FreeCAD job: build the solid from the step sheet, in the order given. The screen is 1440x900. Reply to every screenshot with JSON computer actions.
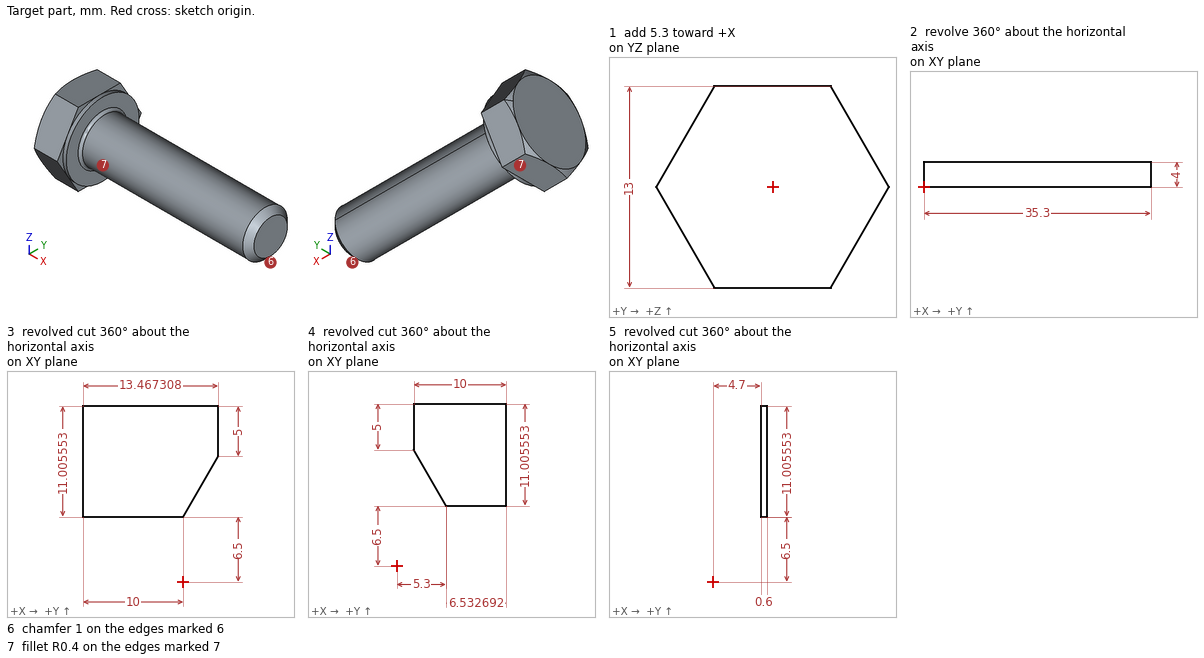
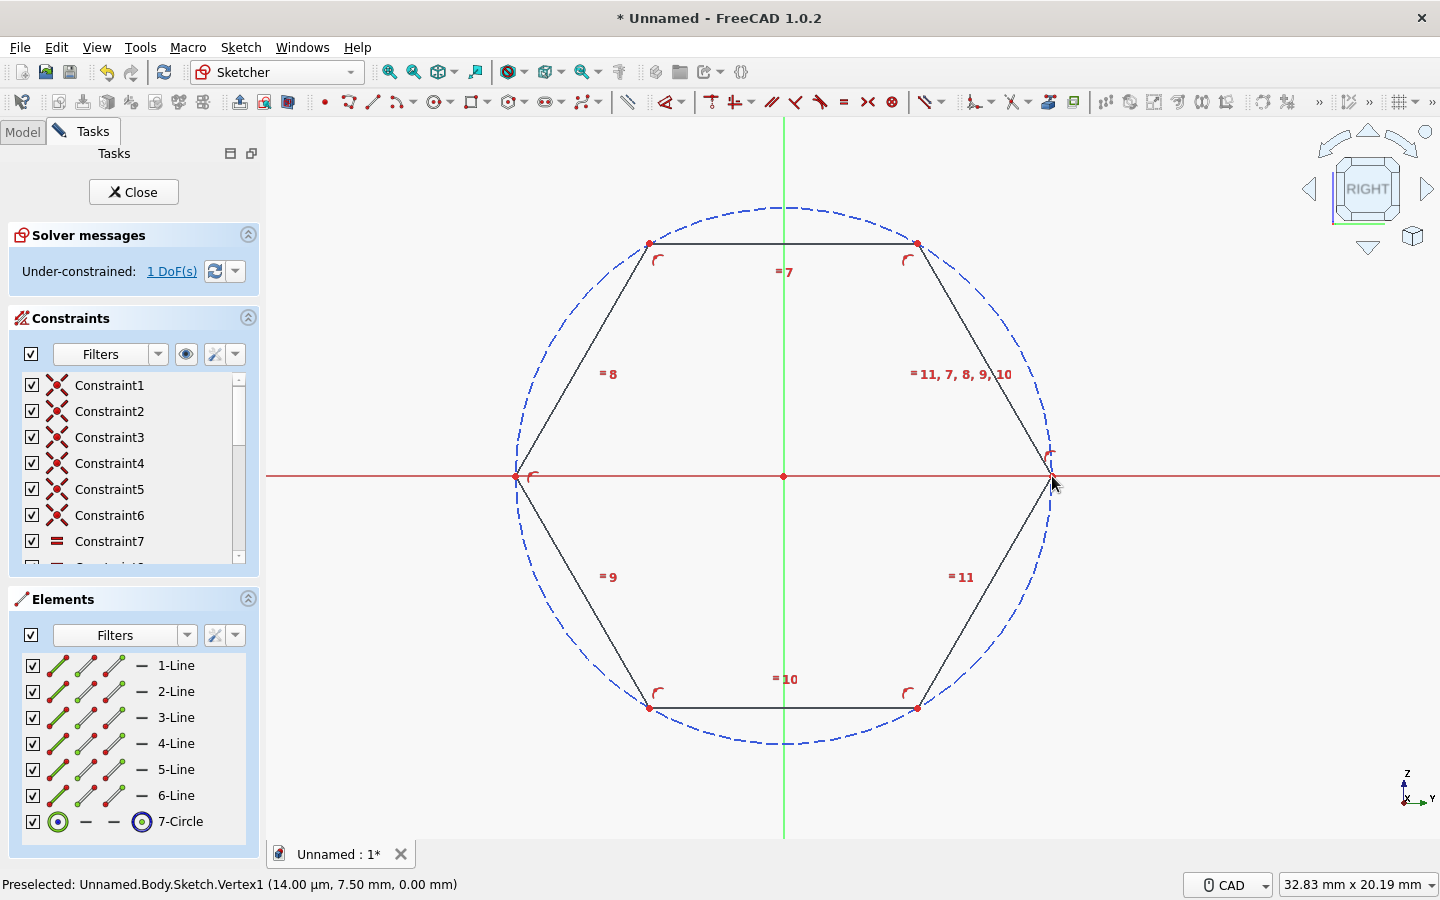
{"action": "key", "text": "d"}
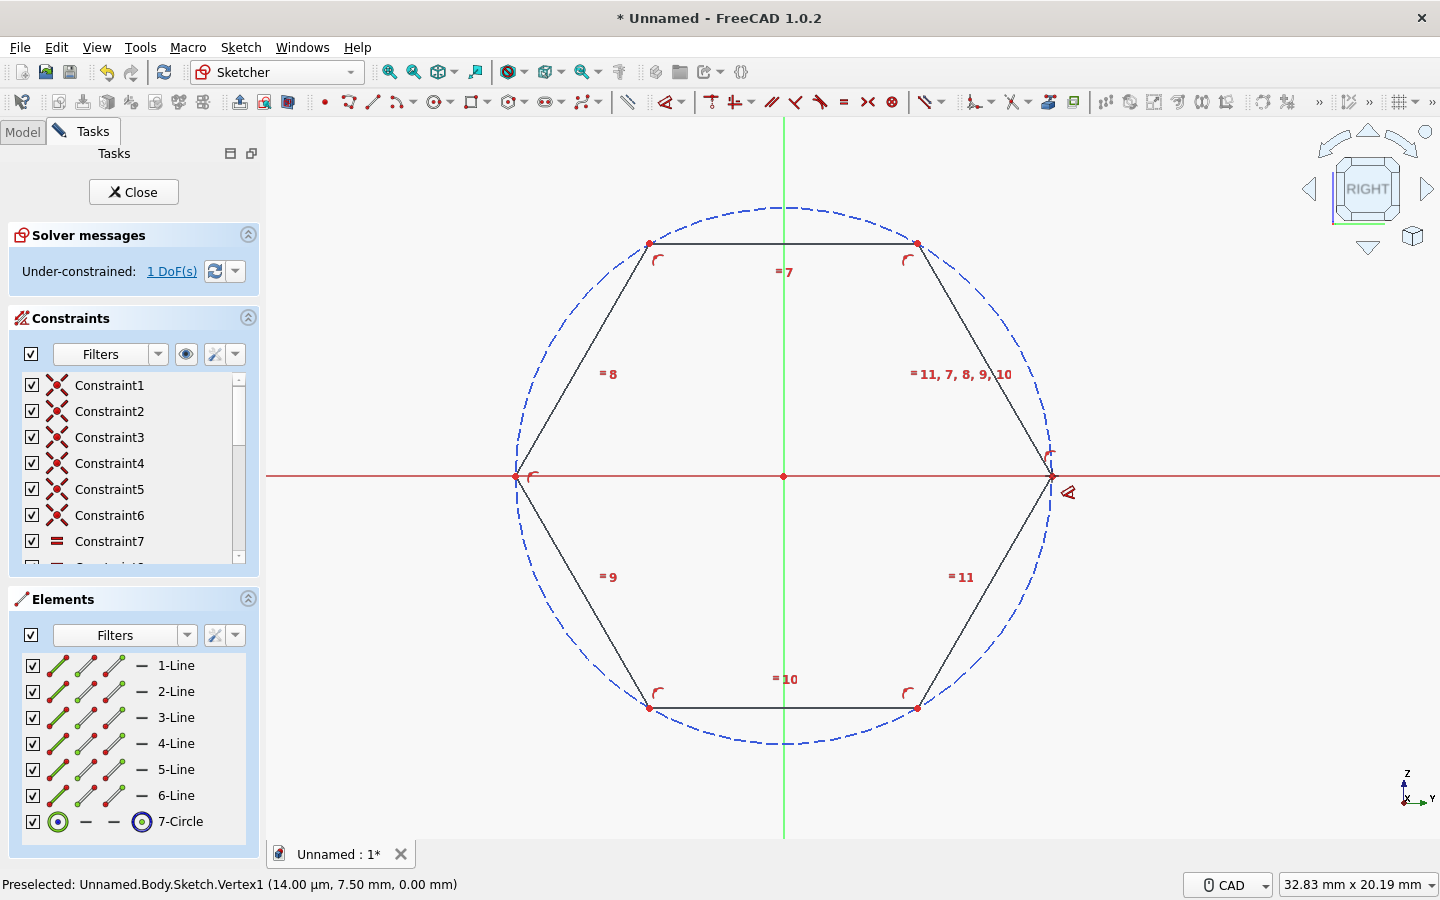
{"action": "left_click", "coordinate": [650, 708]}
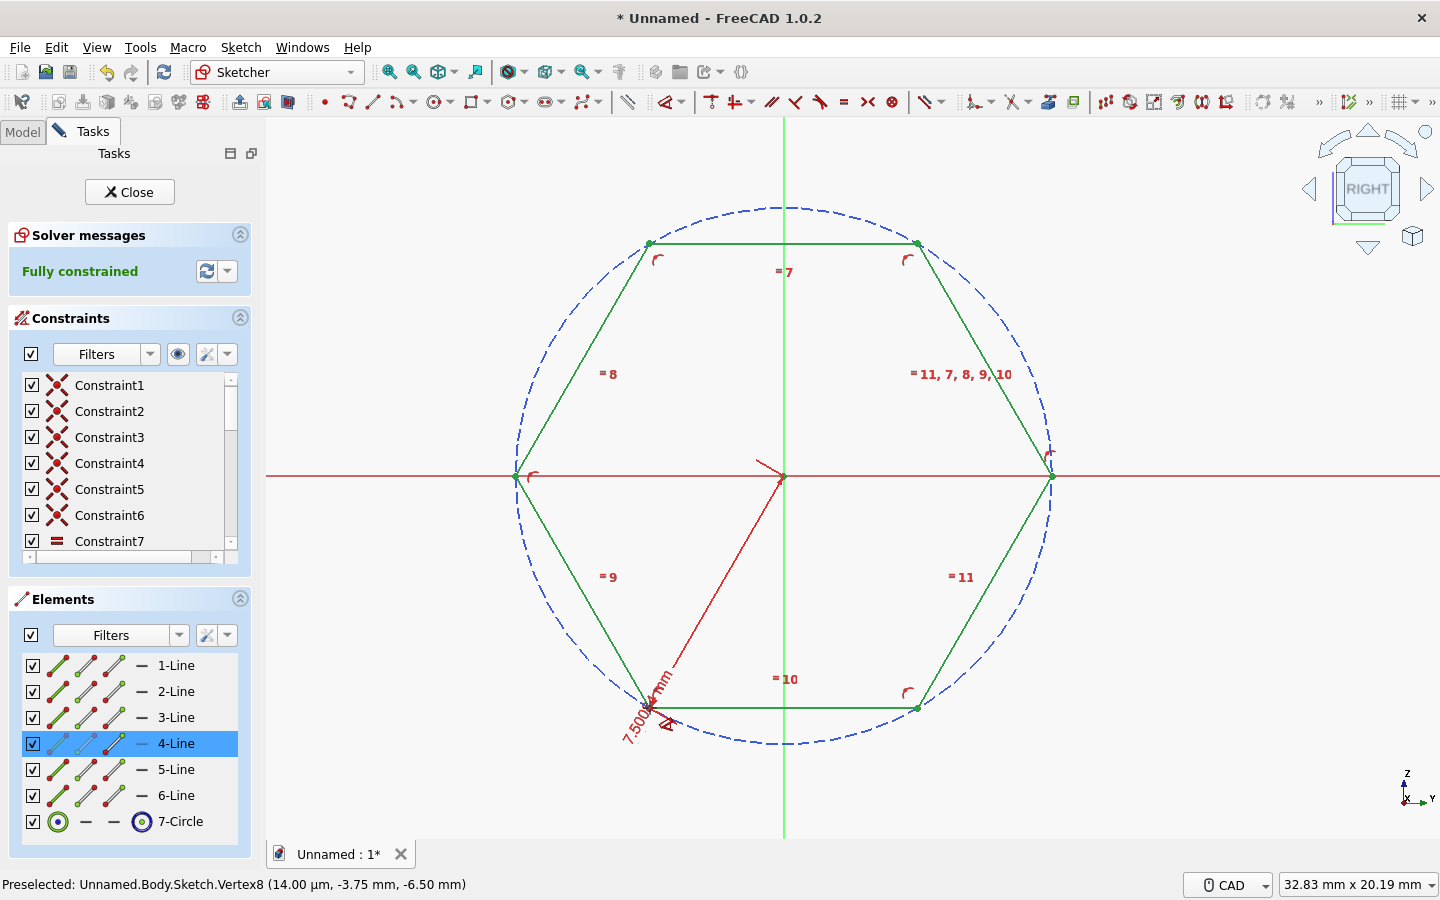
{"action": "left_click", "coordinate": [918, 244]}
{"action": "left_click", "coordinate": [952, 369]}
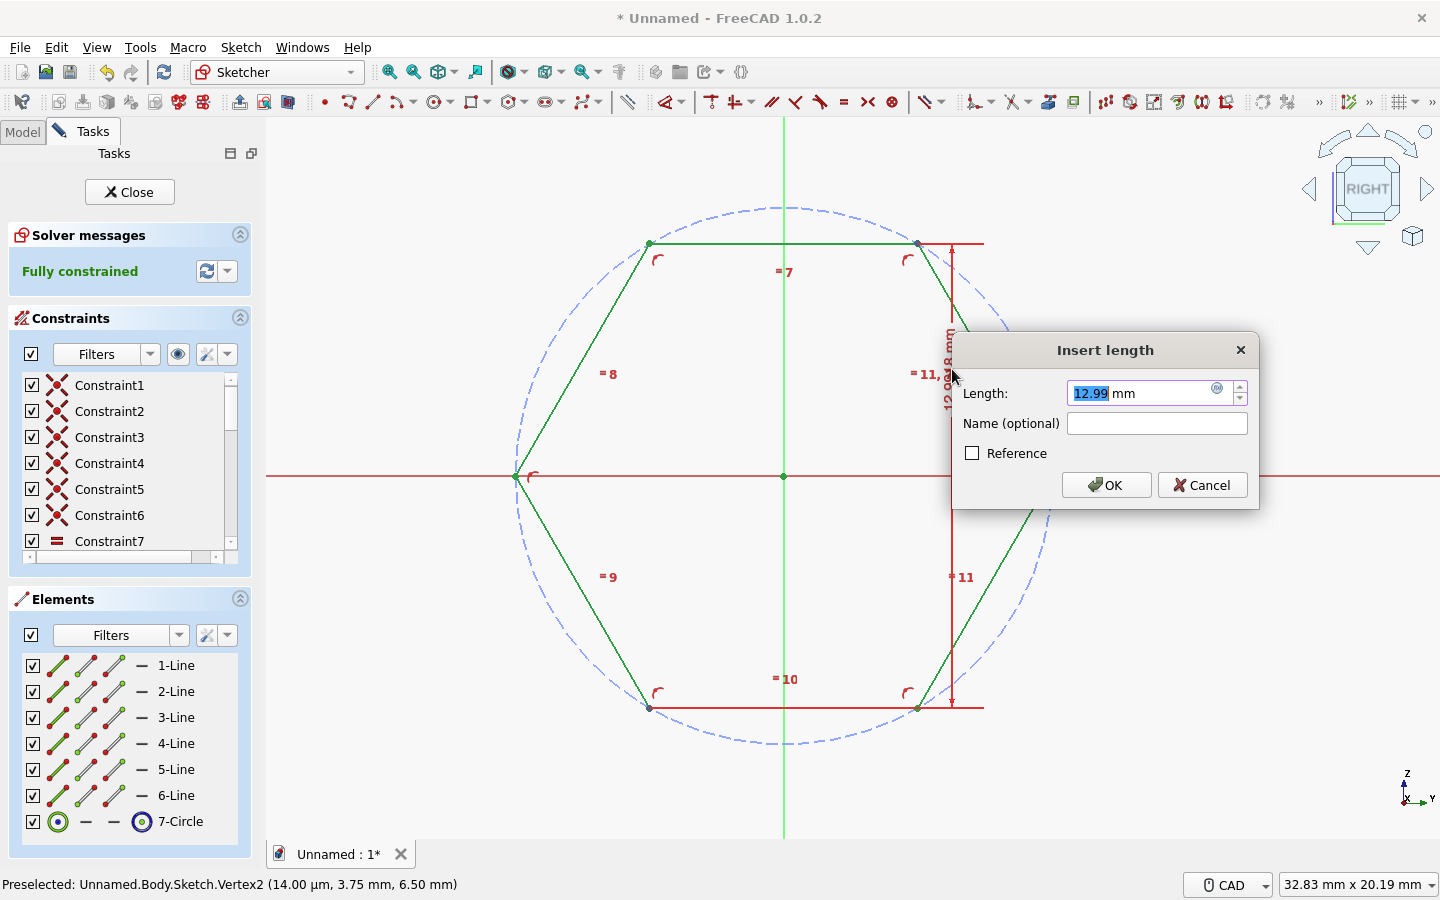
{"action": "type", "text": "13"}
{"action": "key", "text": "Return"}
{"action": "key", "text": "Escape"}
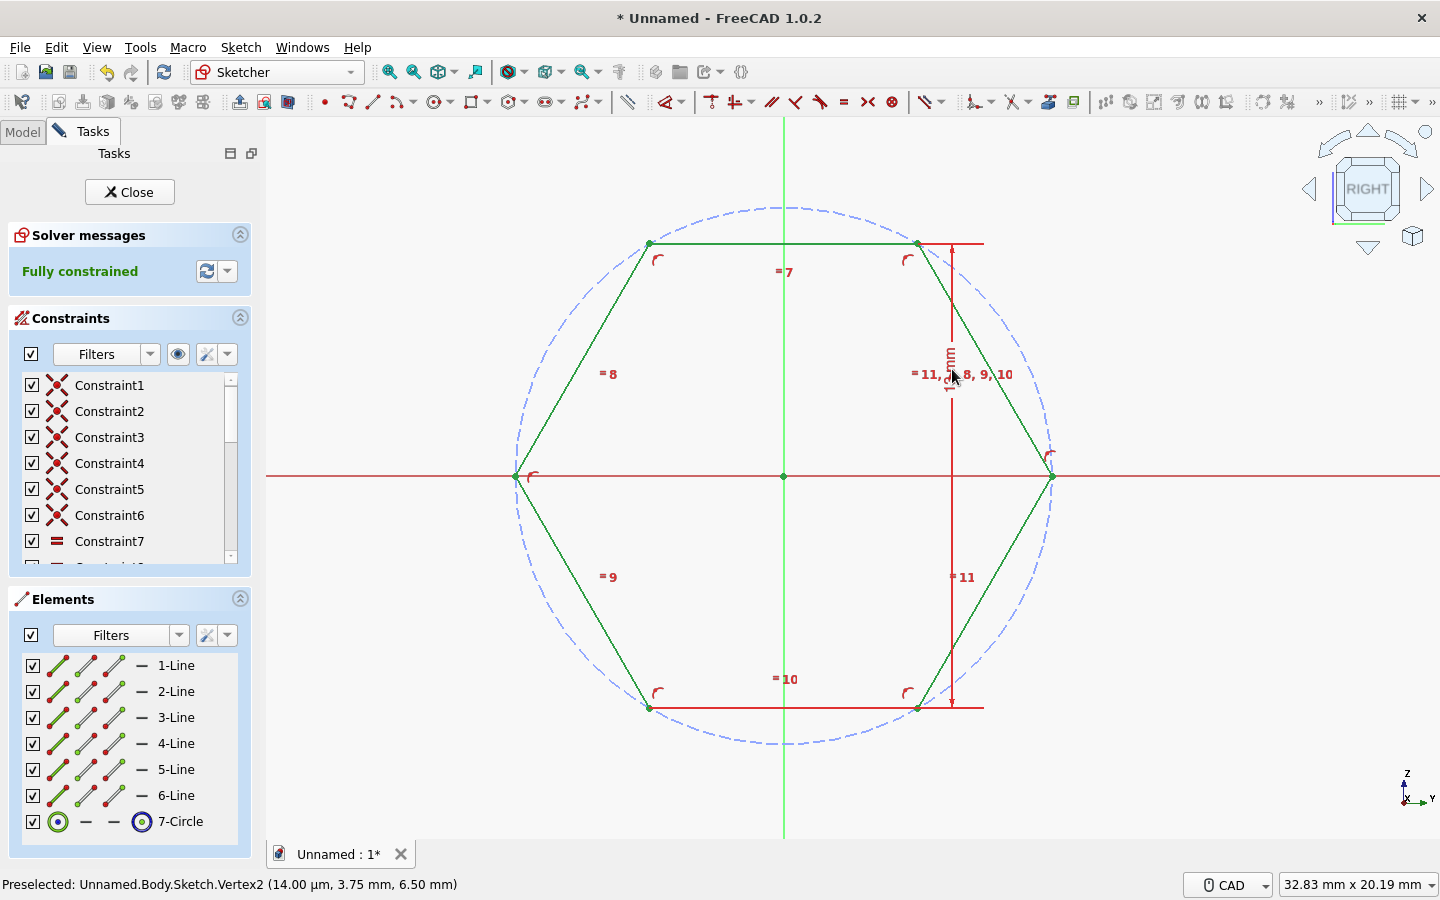
{"action": "left_click", "coordinate": [130, 192]}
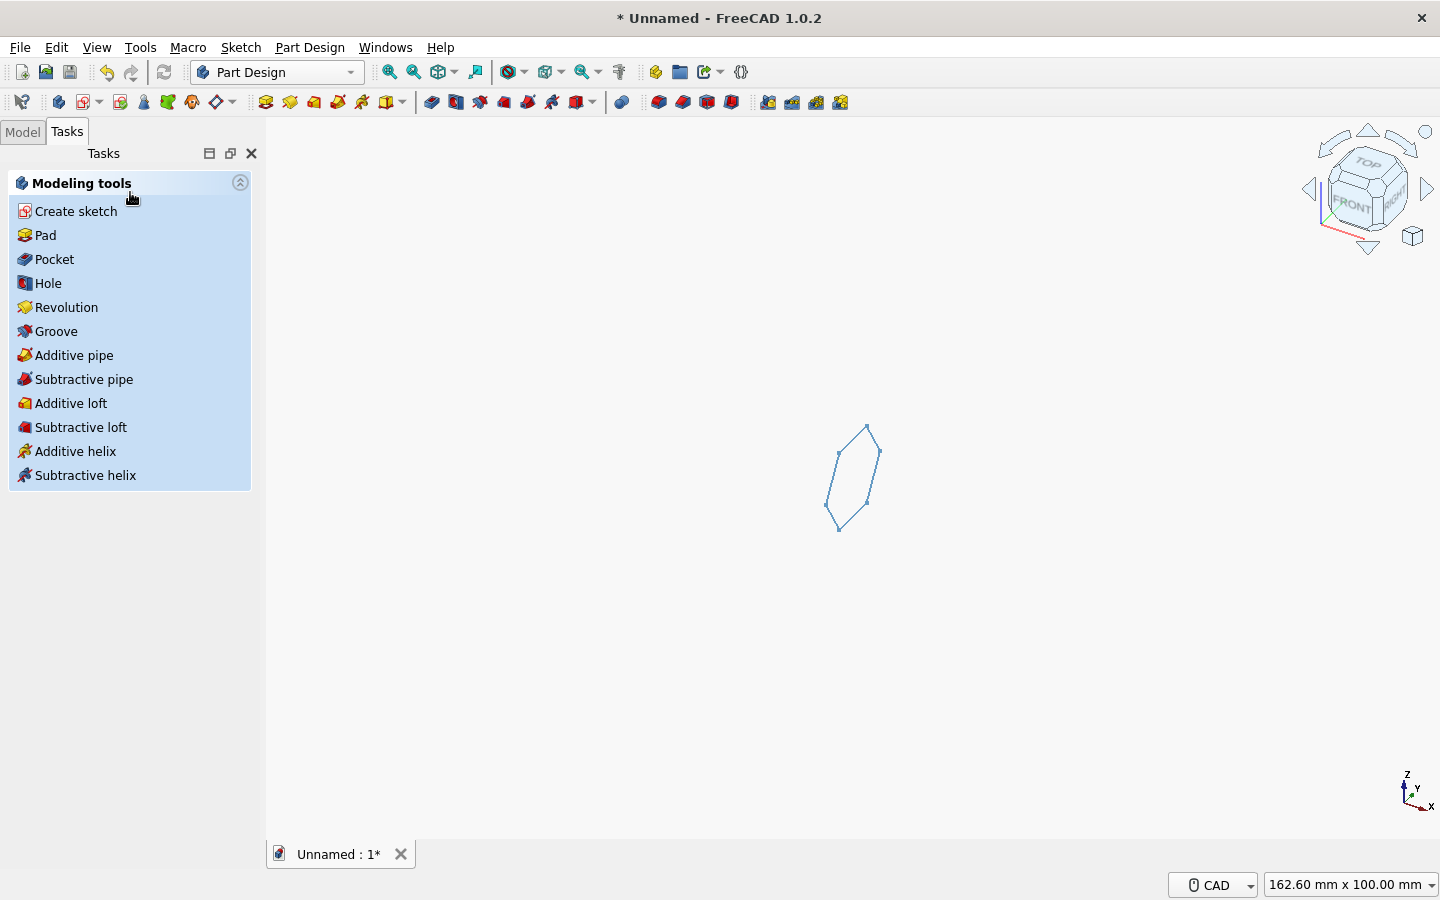
{"action": "left_click", "coordinate": [266, 102]}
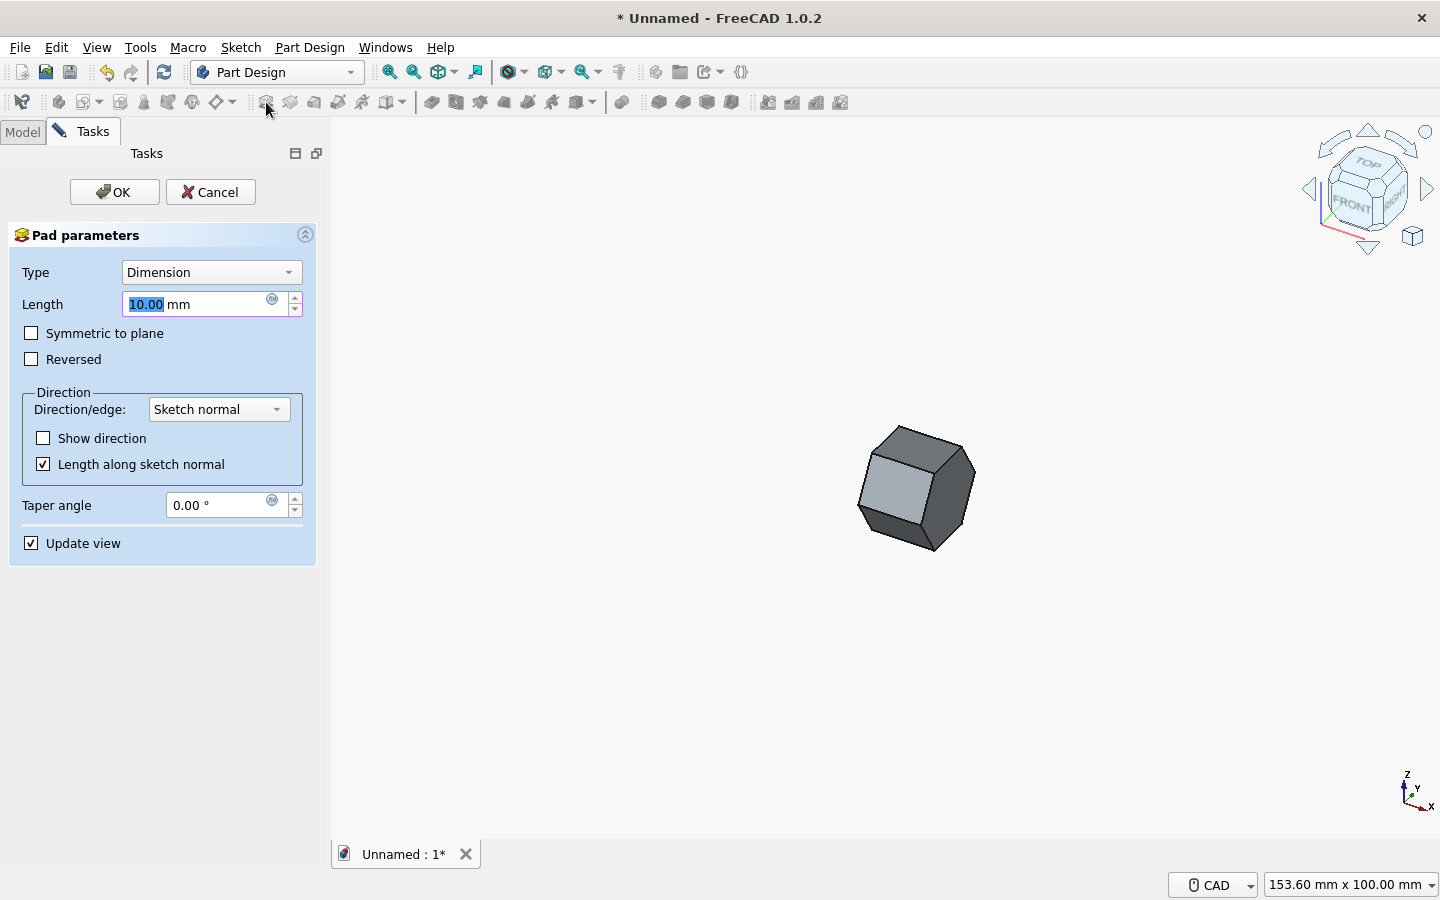
{"action": "type", "text": "5.3"}
{"action": "key", "text": "Tab"}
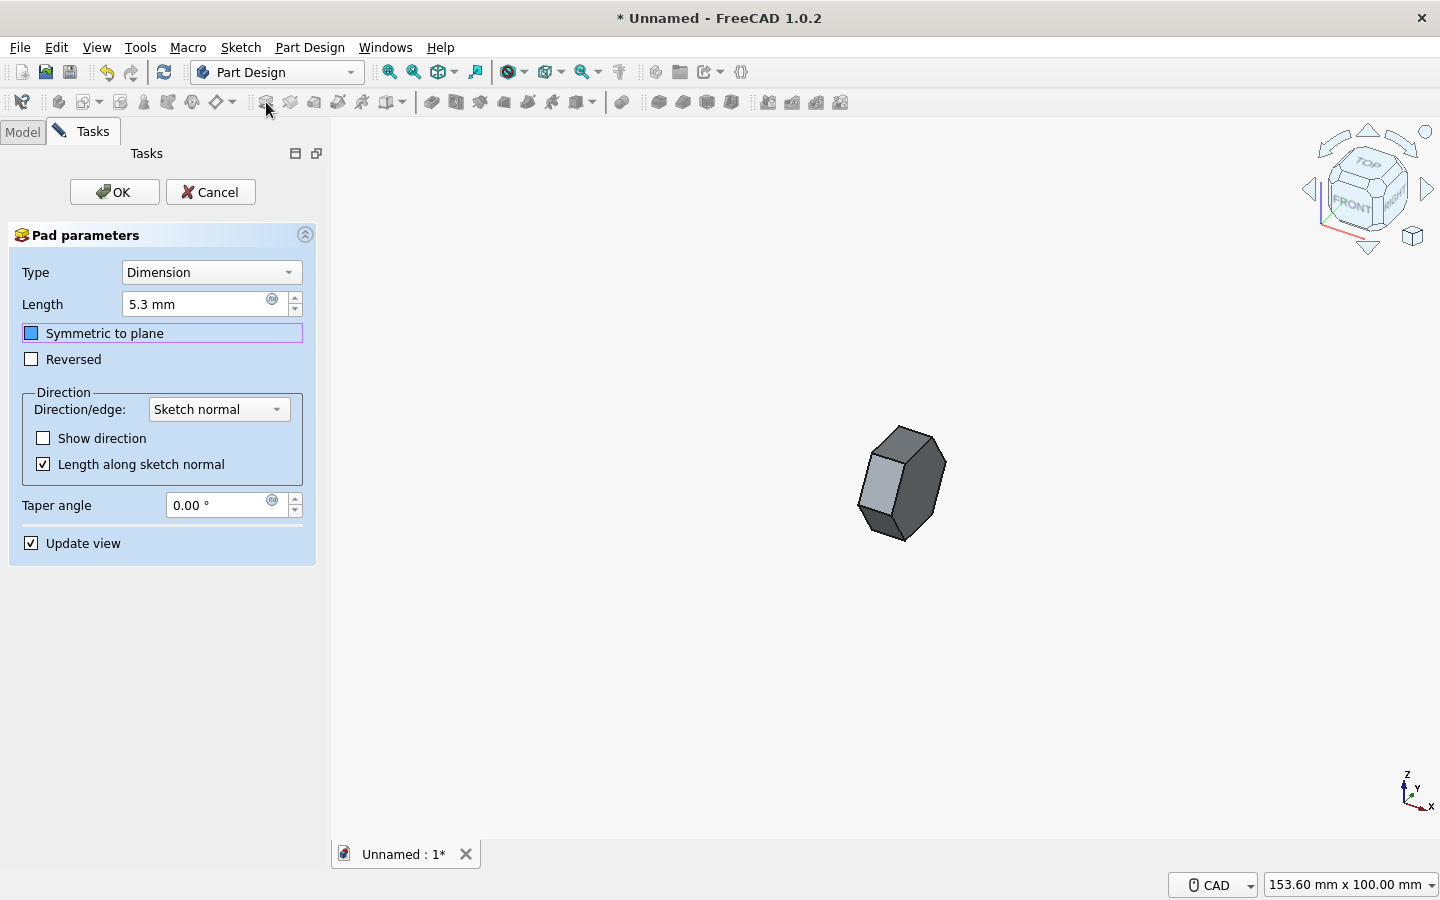
{"action": "left_click", "coordinate": [115, 192]}